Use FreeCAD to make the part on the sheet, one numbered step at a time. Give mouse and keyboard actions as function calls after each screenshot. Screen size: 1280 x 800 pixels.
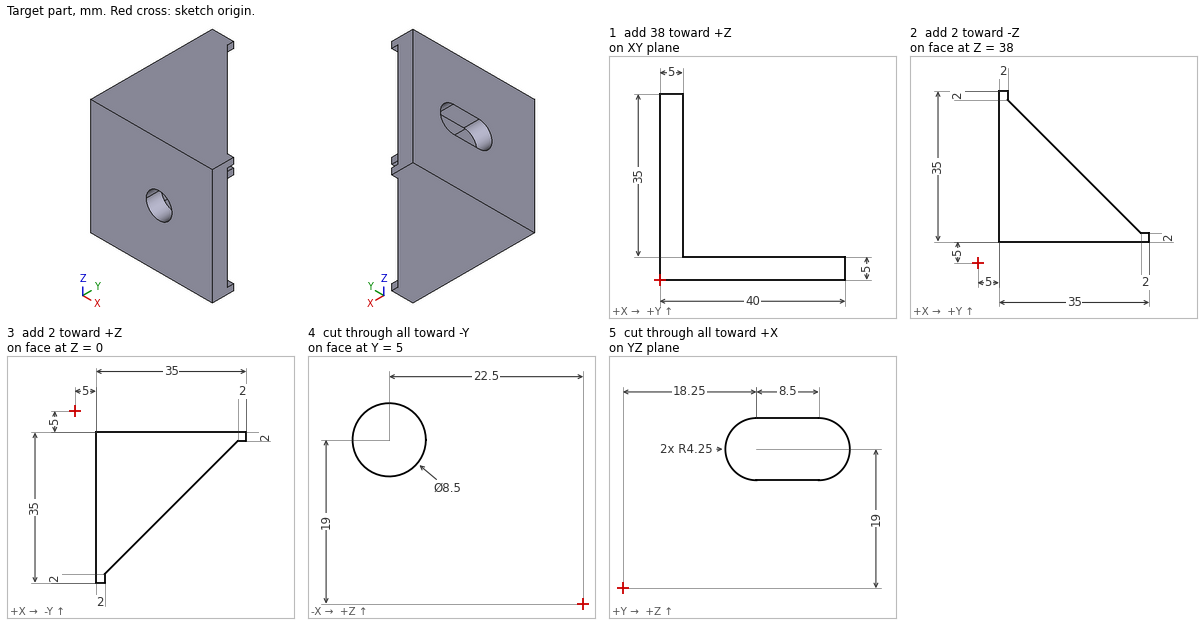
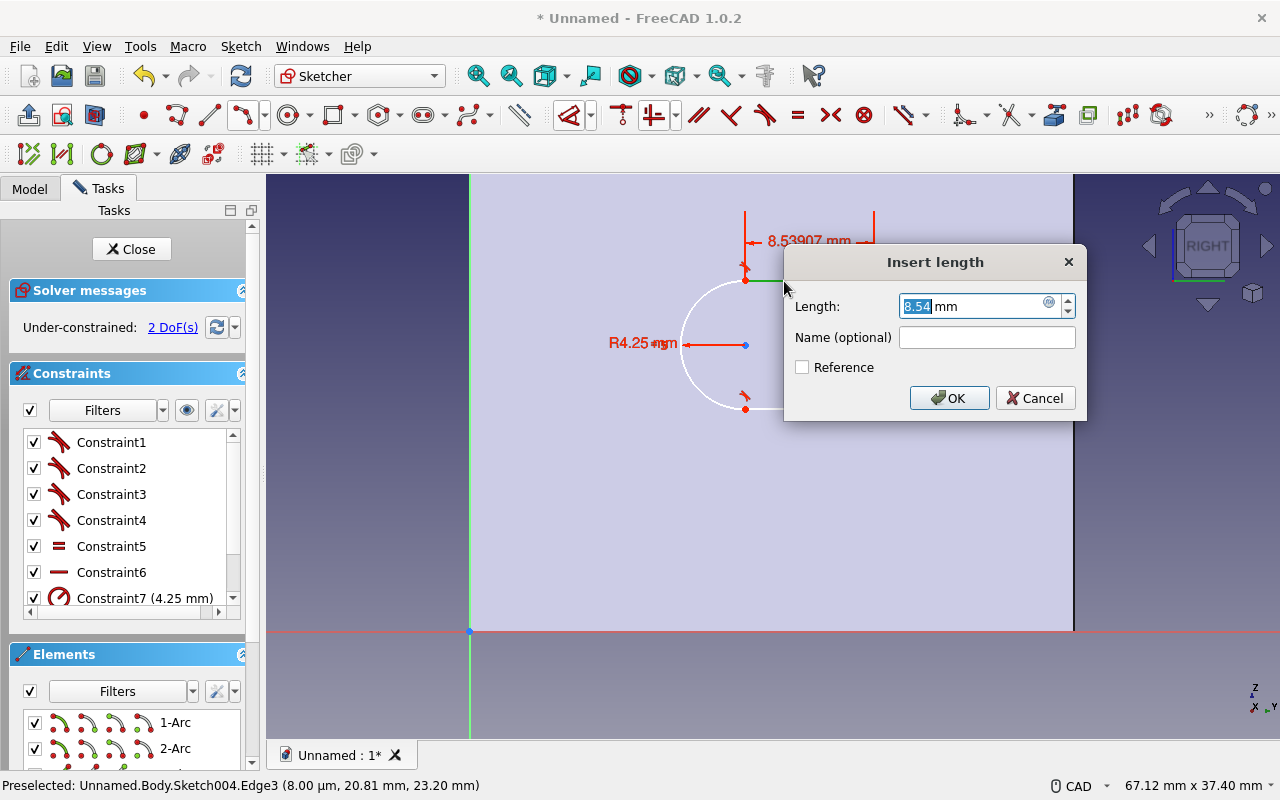
text(8.5)
key(Return)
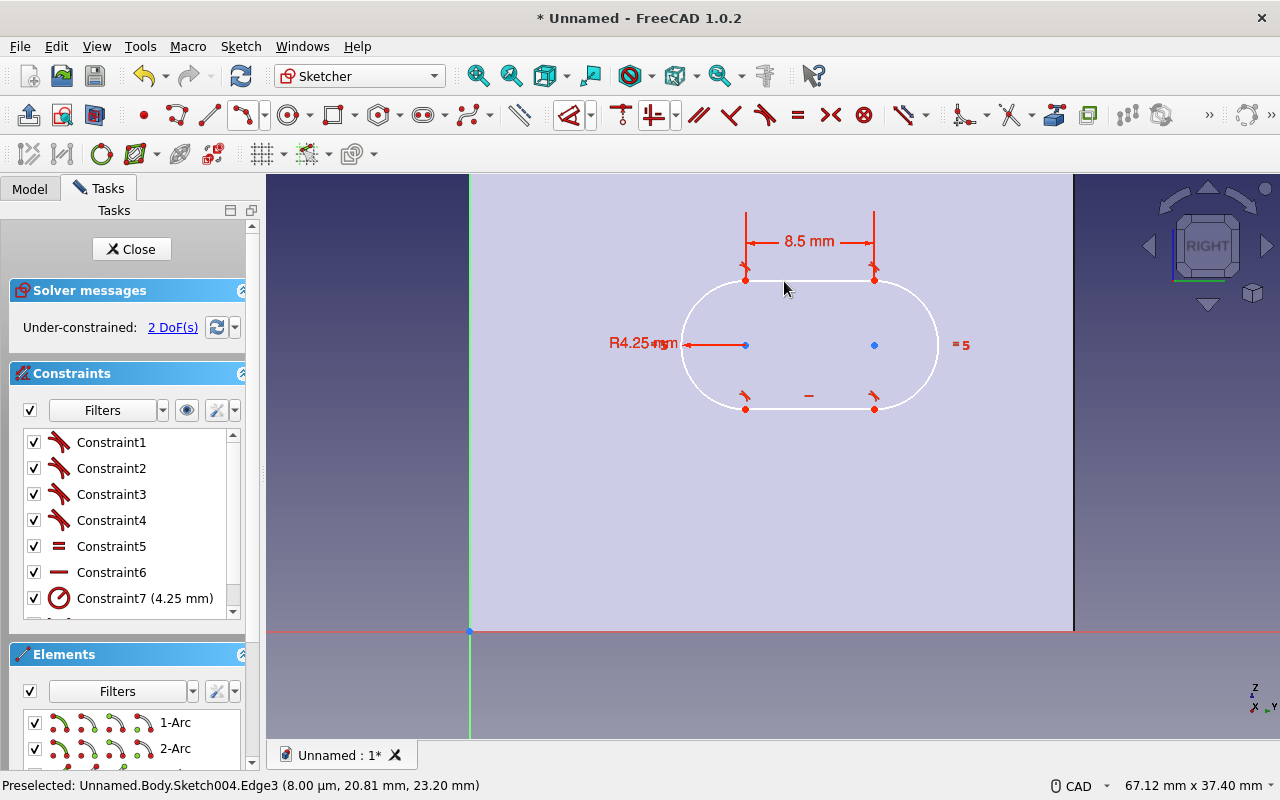
click(746, 345)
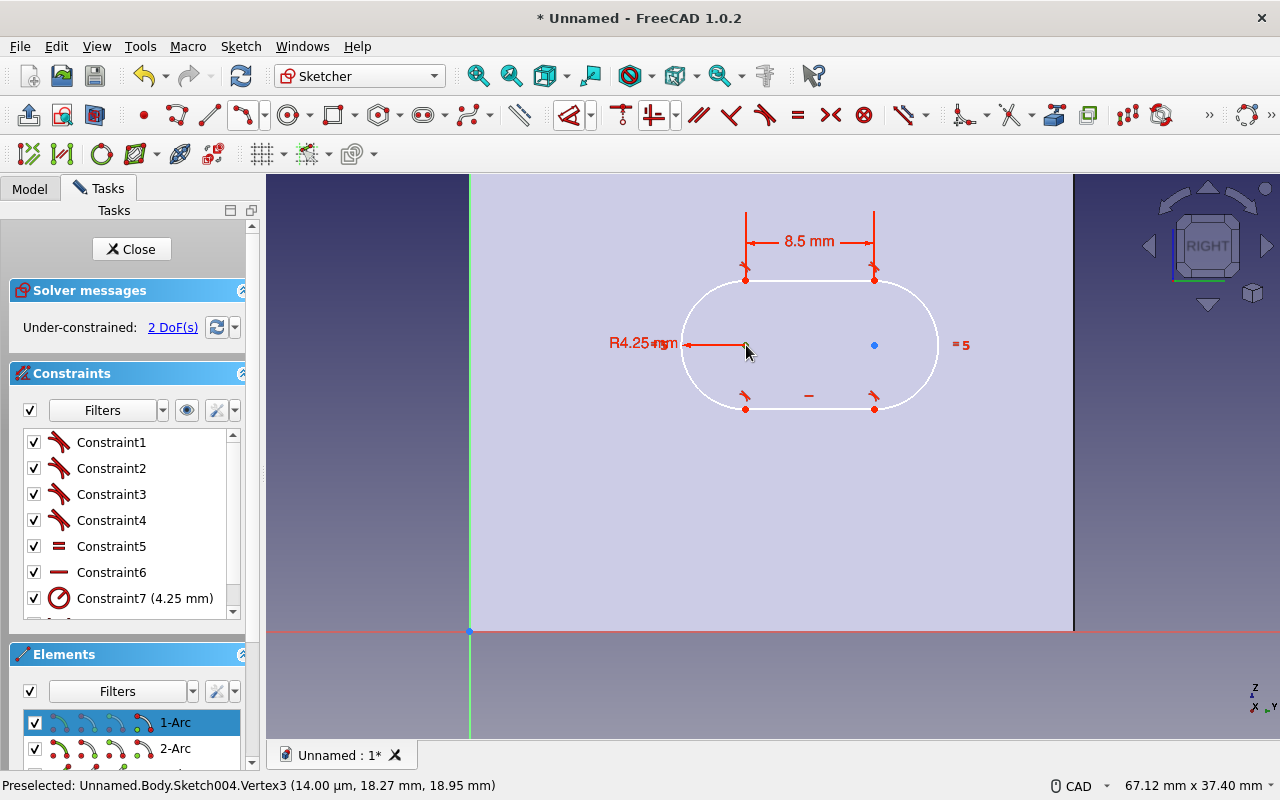
key(i)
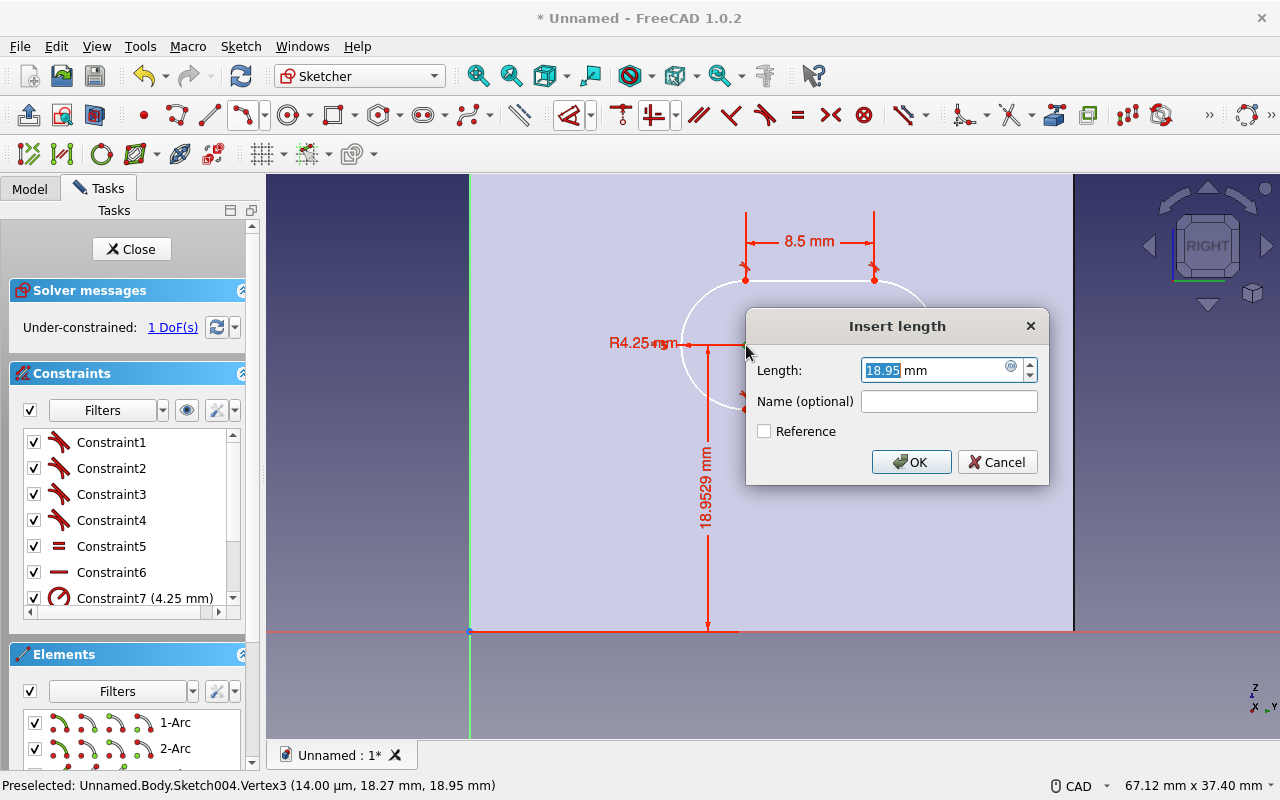
text(19)
key(Return)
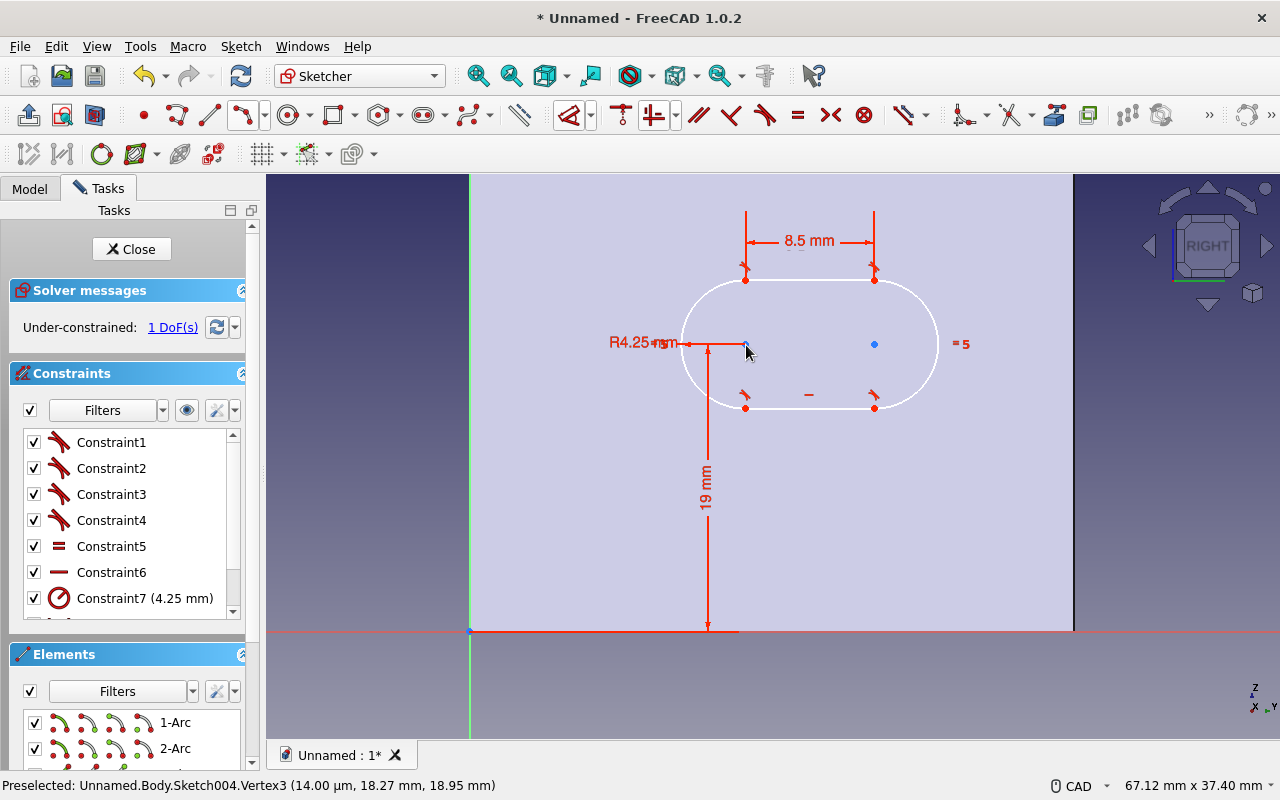
click(746, 280)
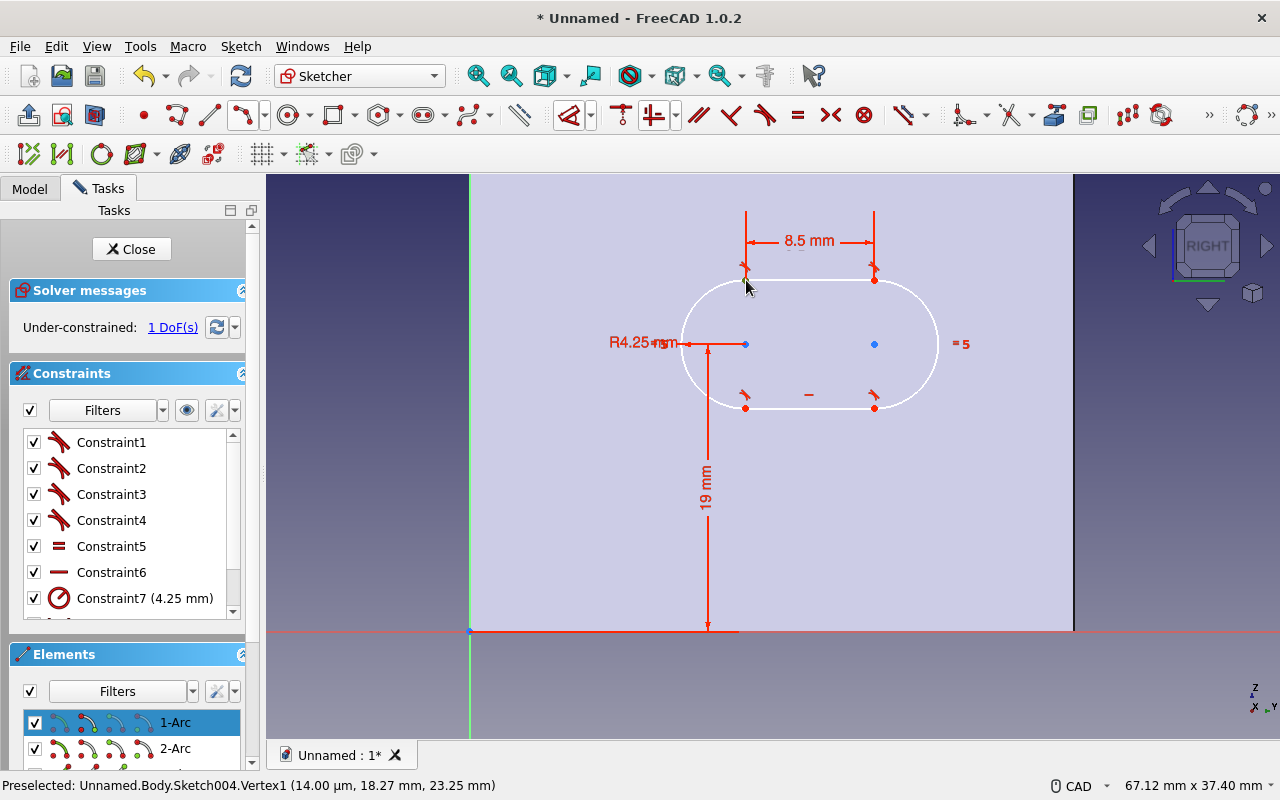
key(l)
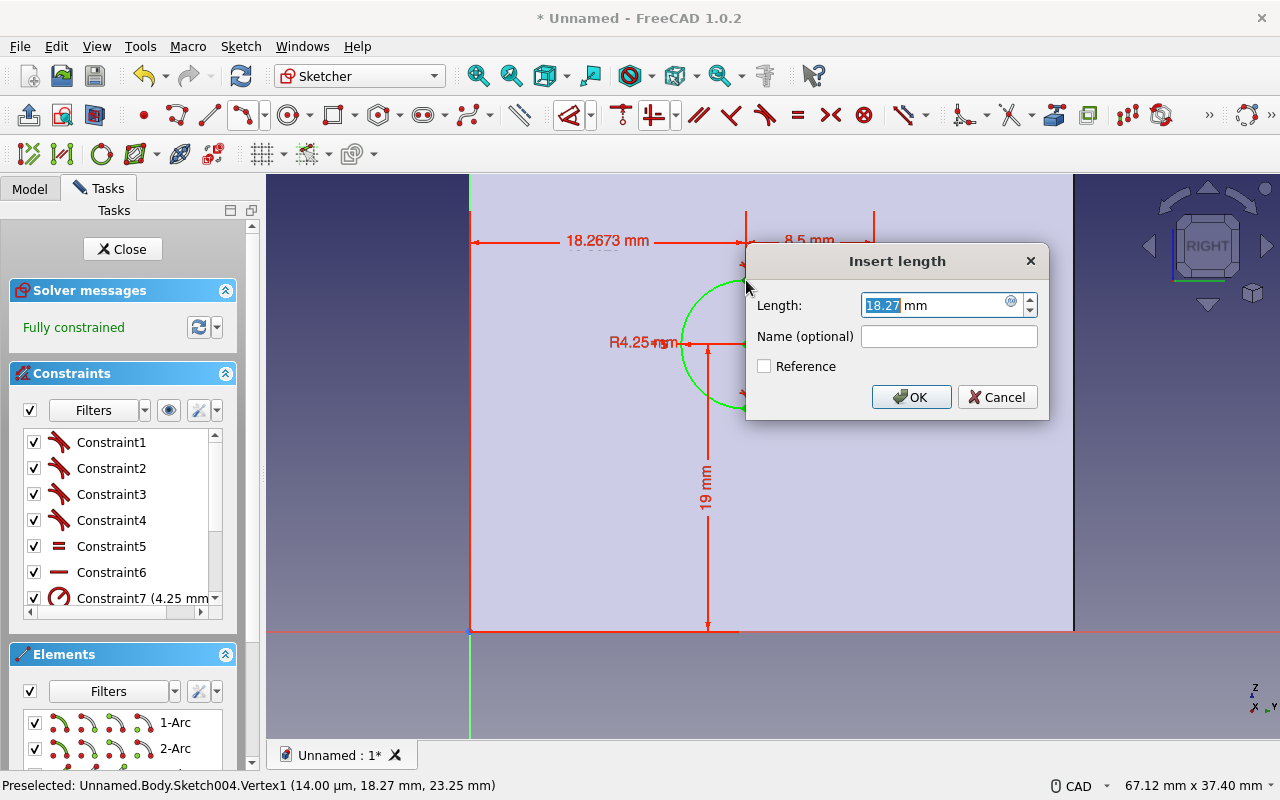
text(18.25)
key(Return)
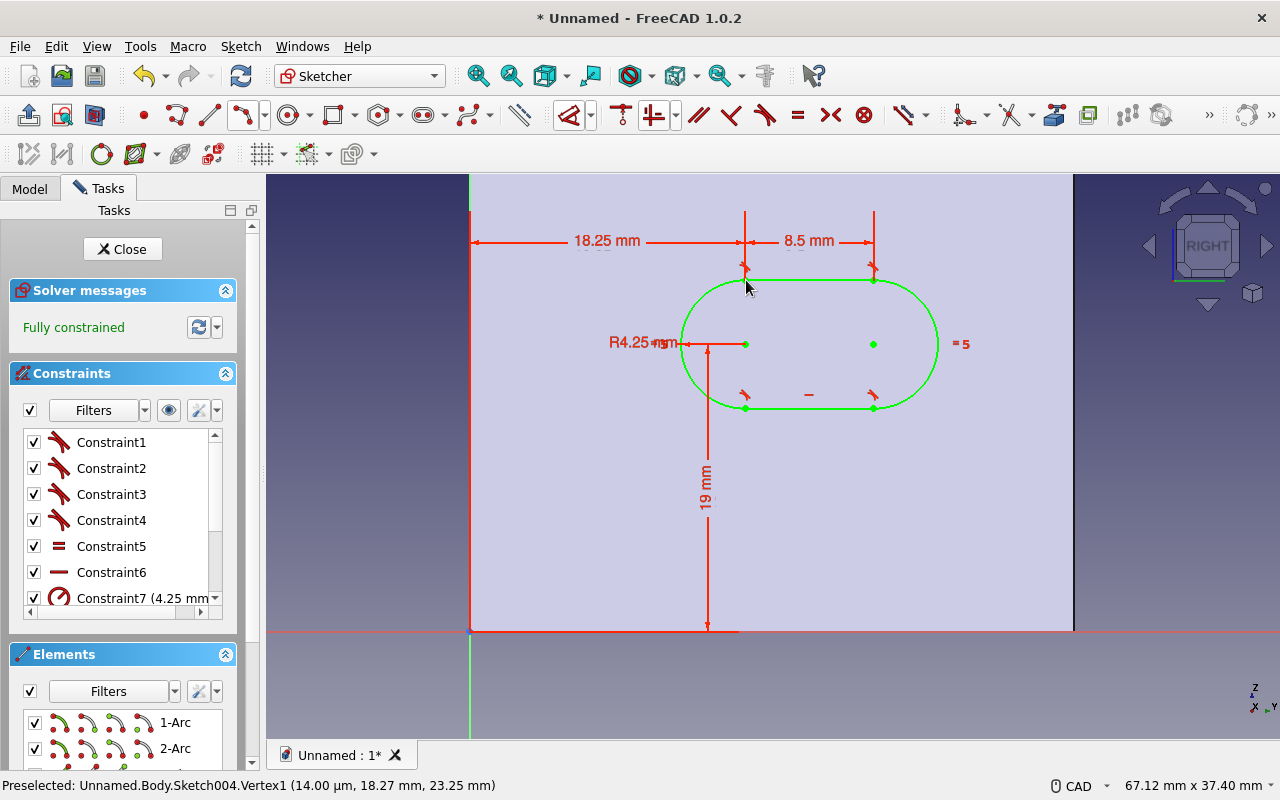
click(123, 249)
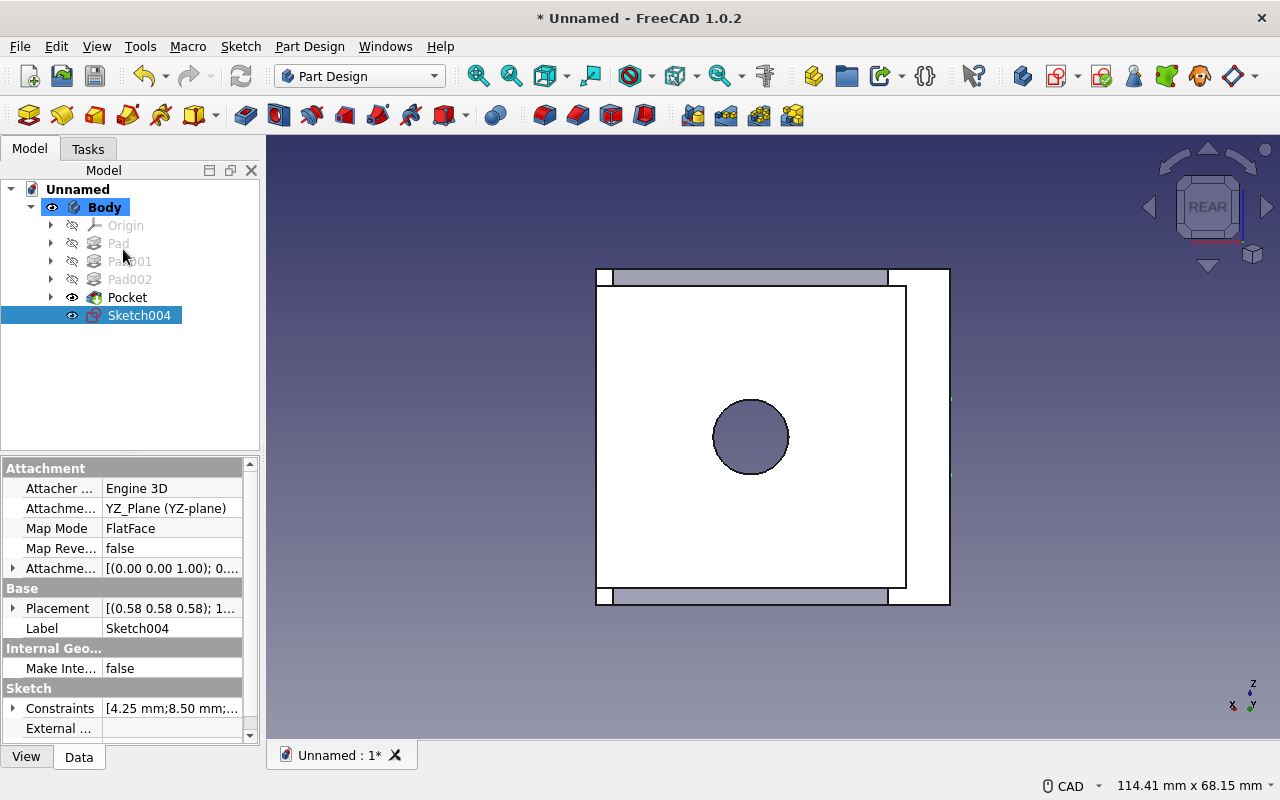
click(246, 116)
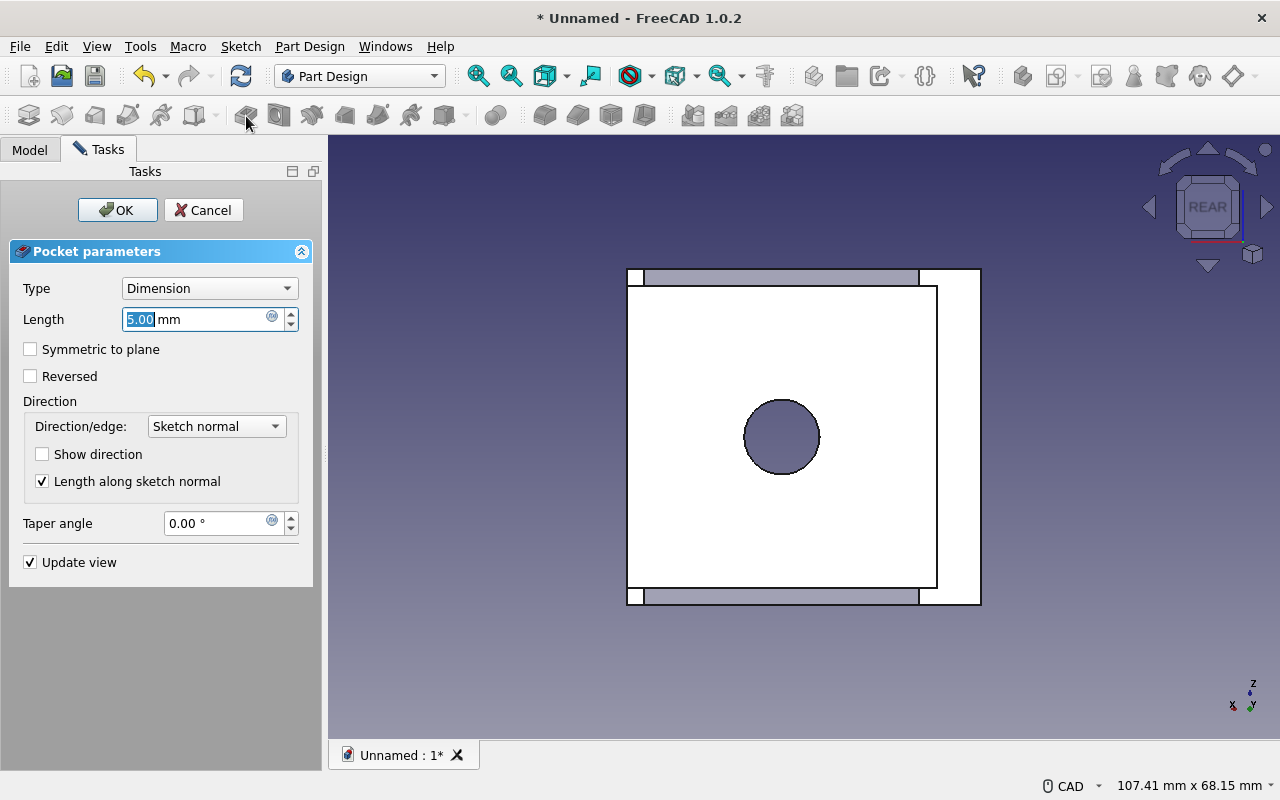
click(210, 288)